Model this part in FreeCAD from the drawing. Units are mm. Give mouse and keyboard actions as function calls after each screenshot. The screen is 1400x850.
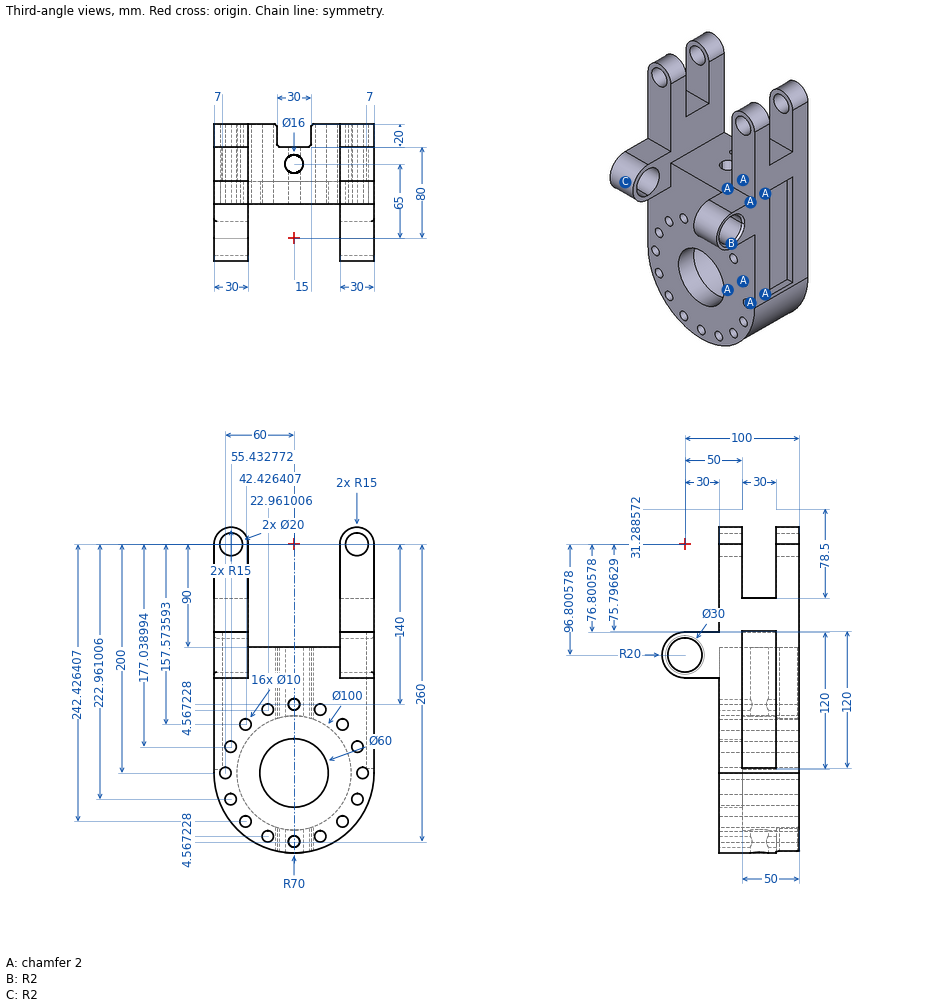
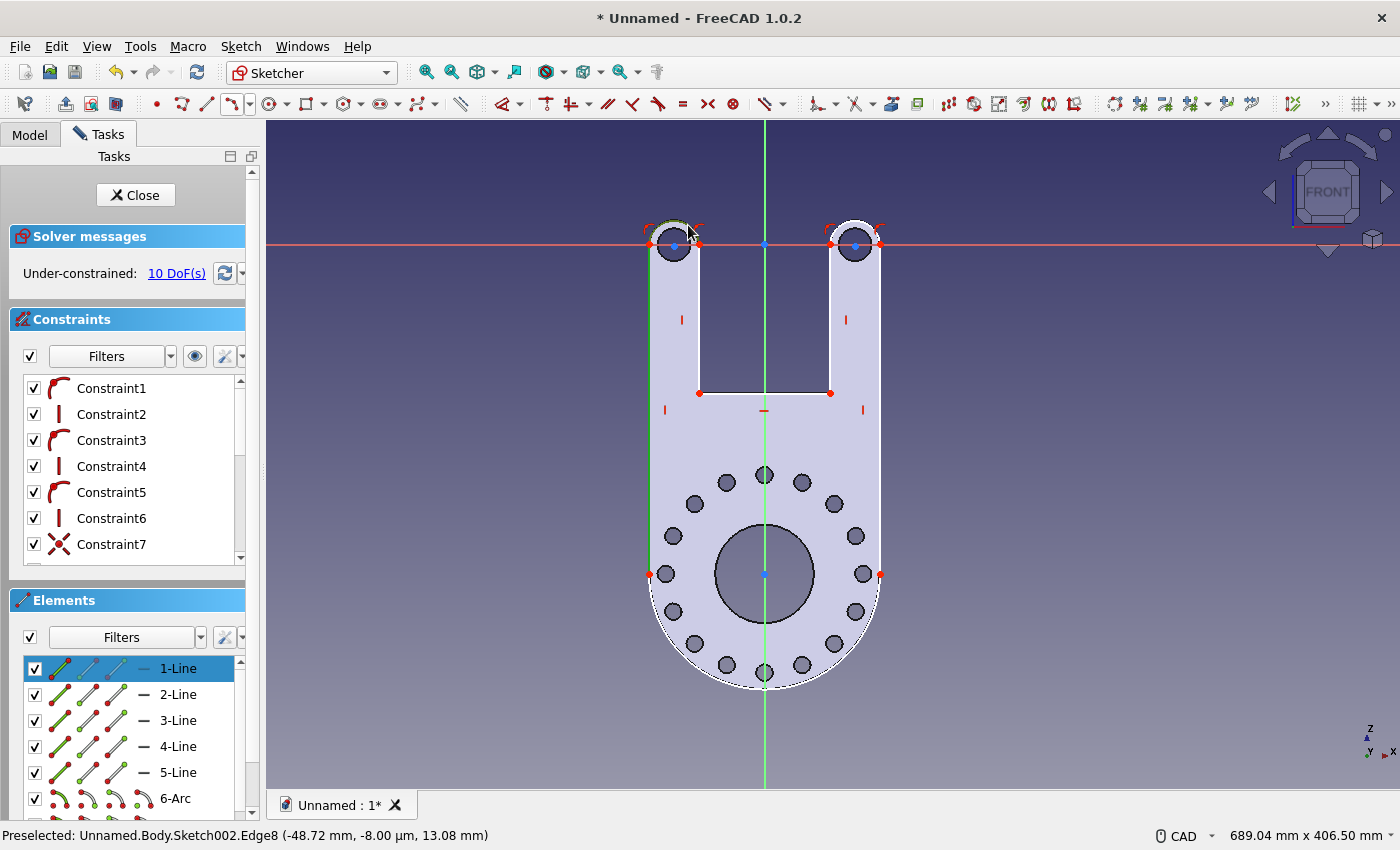
key(t)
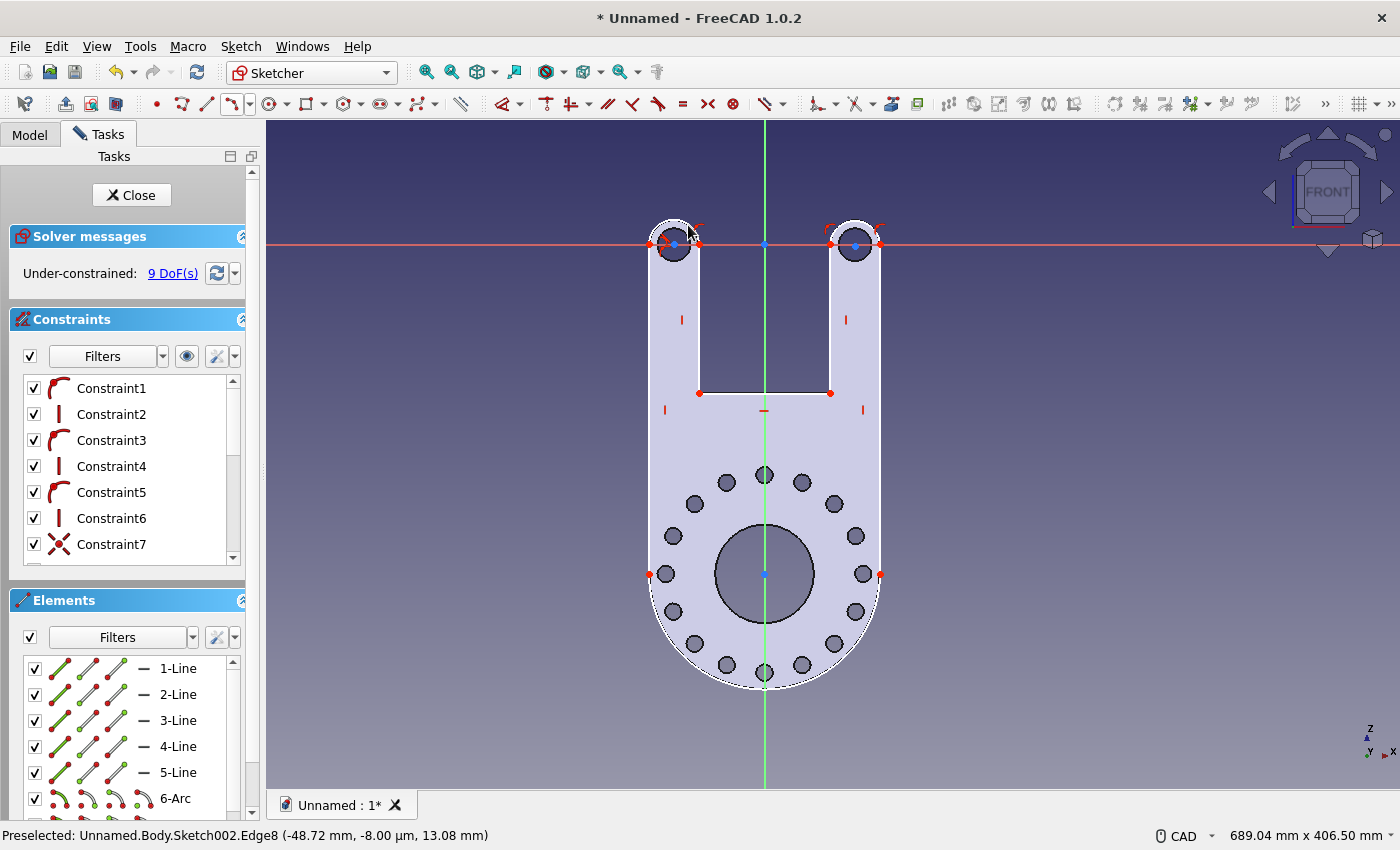
click(880, 476)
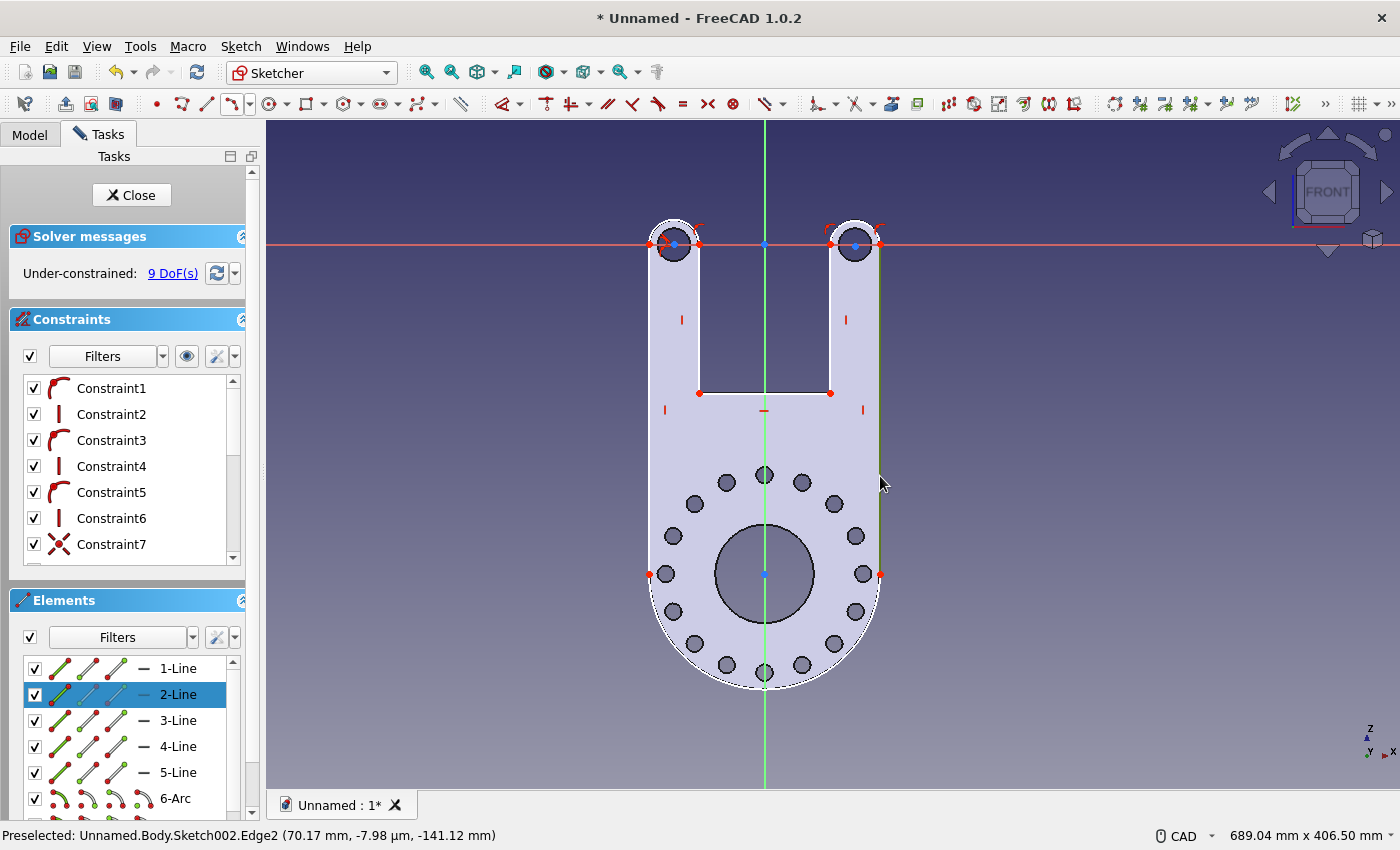
click(869, 225)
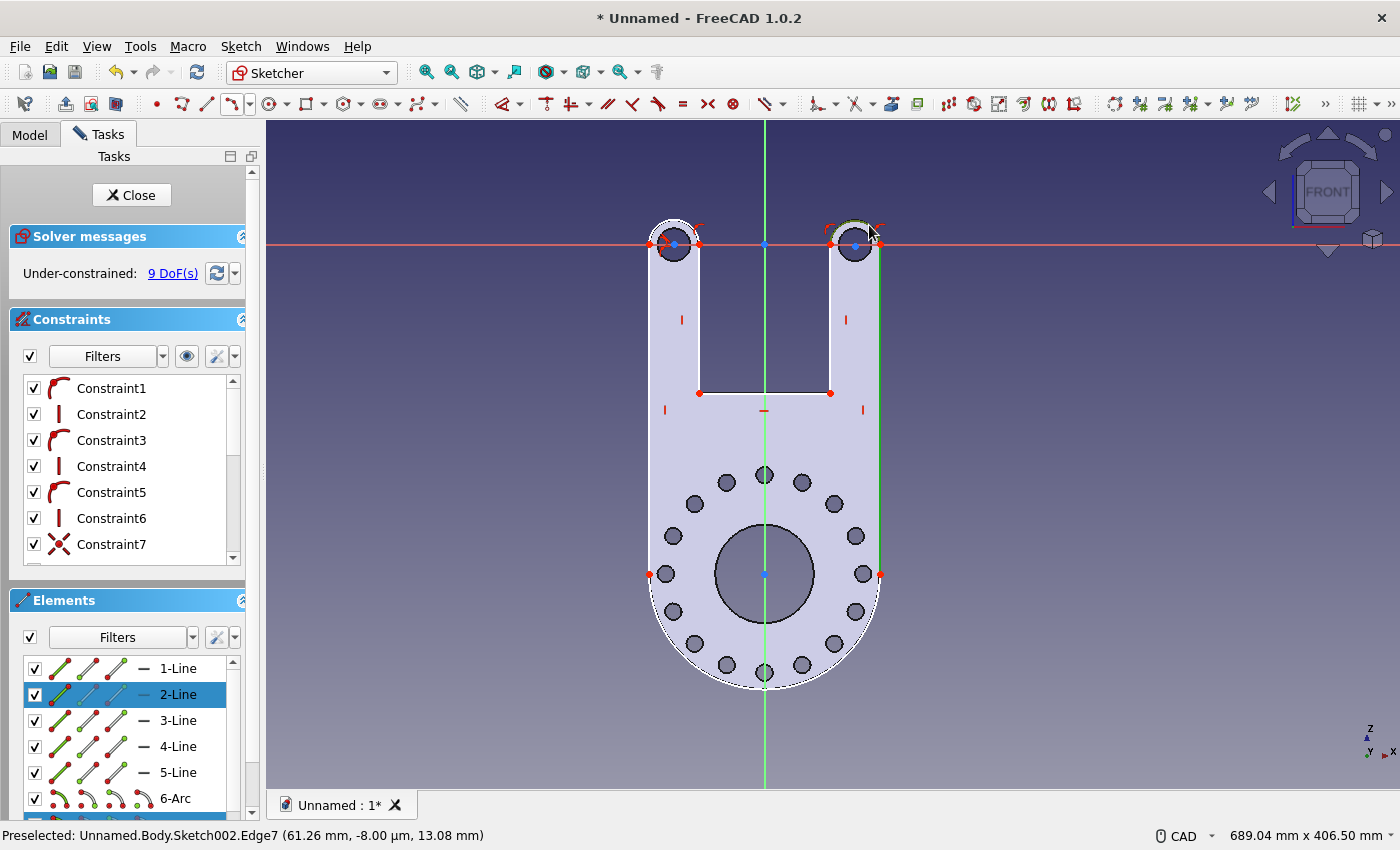
key(t)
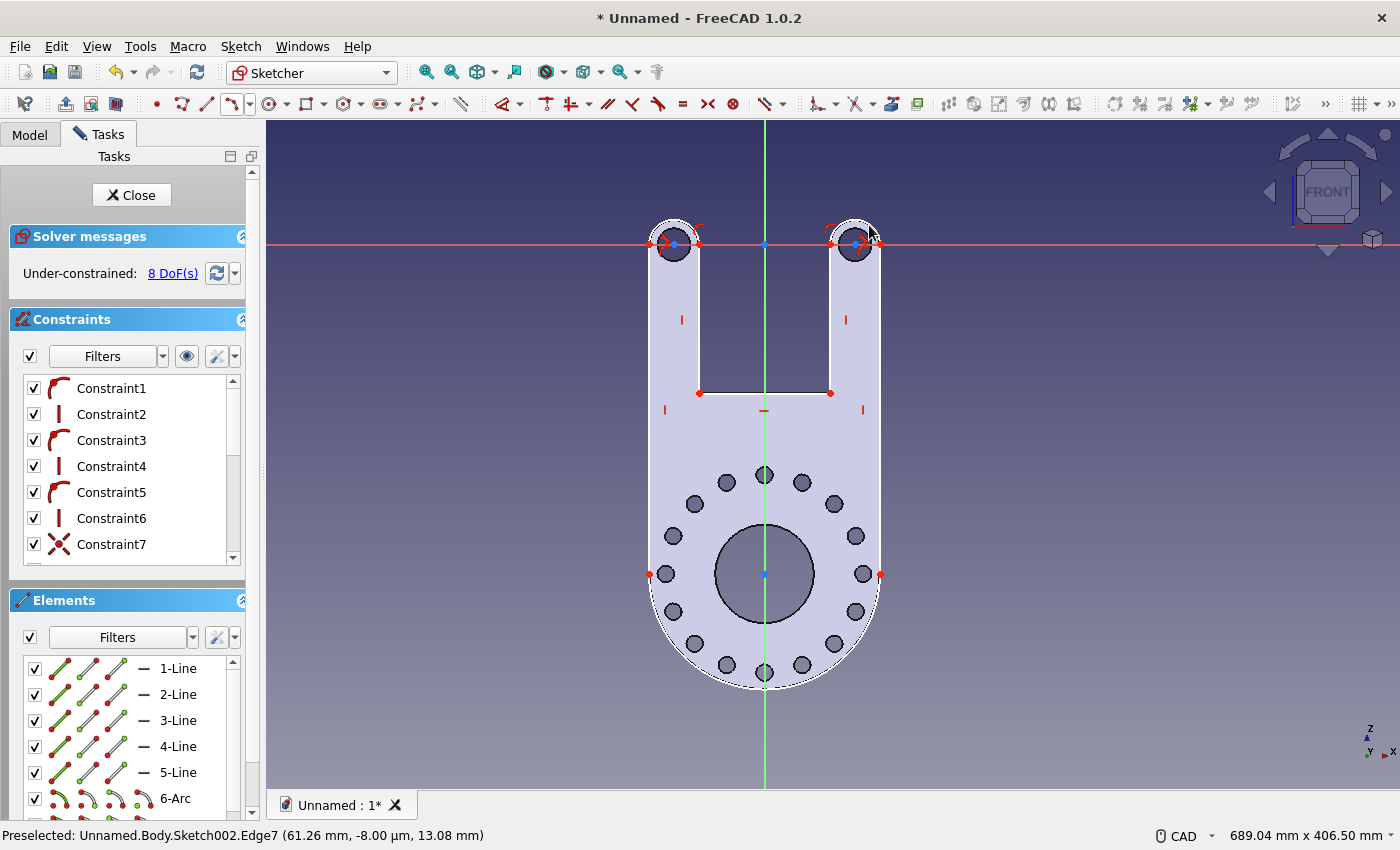
click(870, 225)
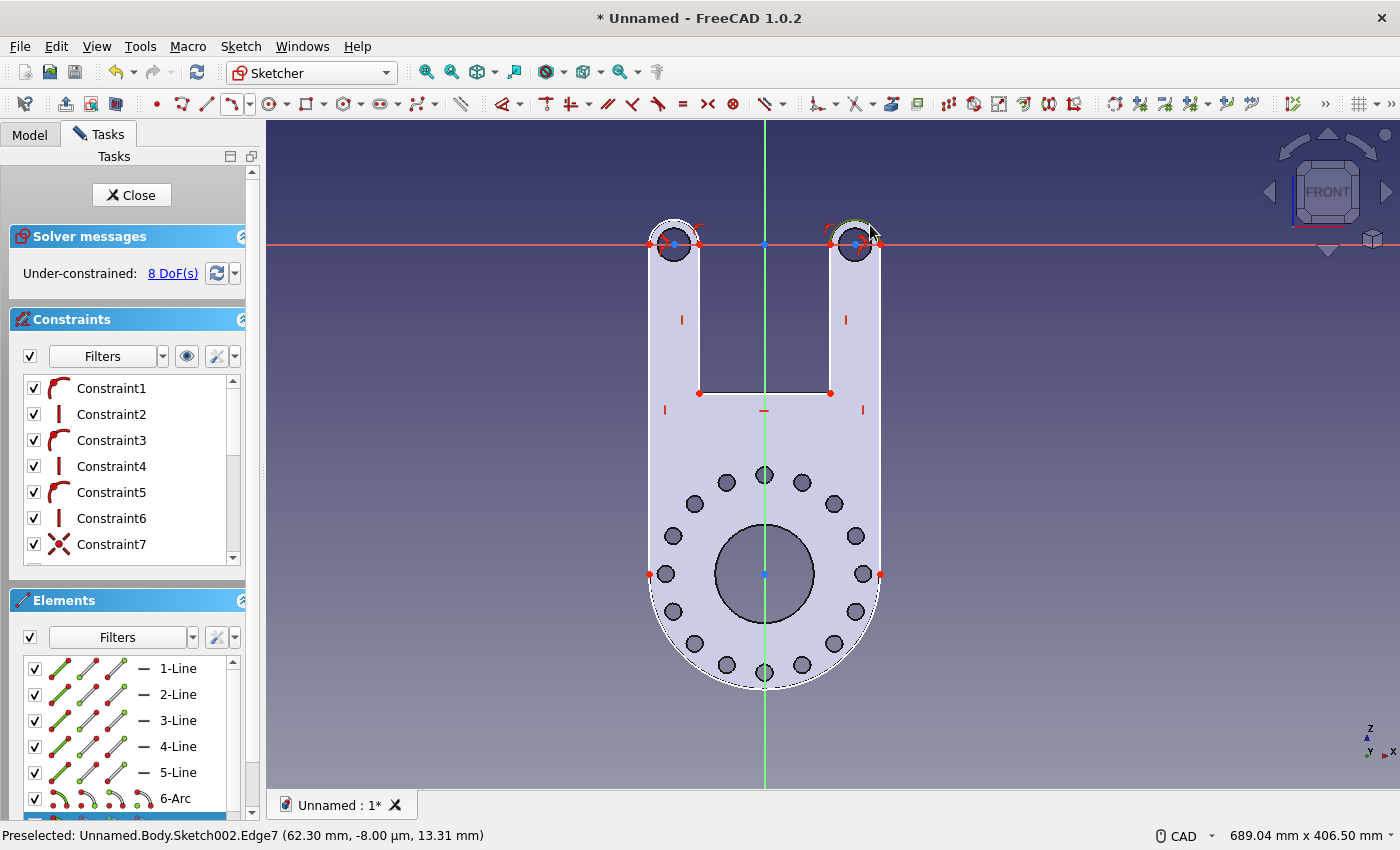
click(689, 225)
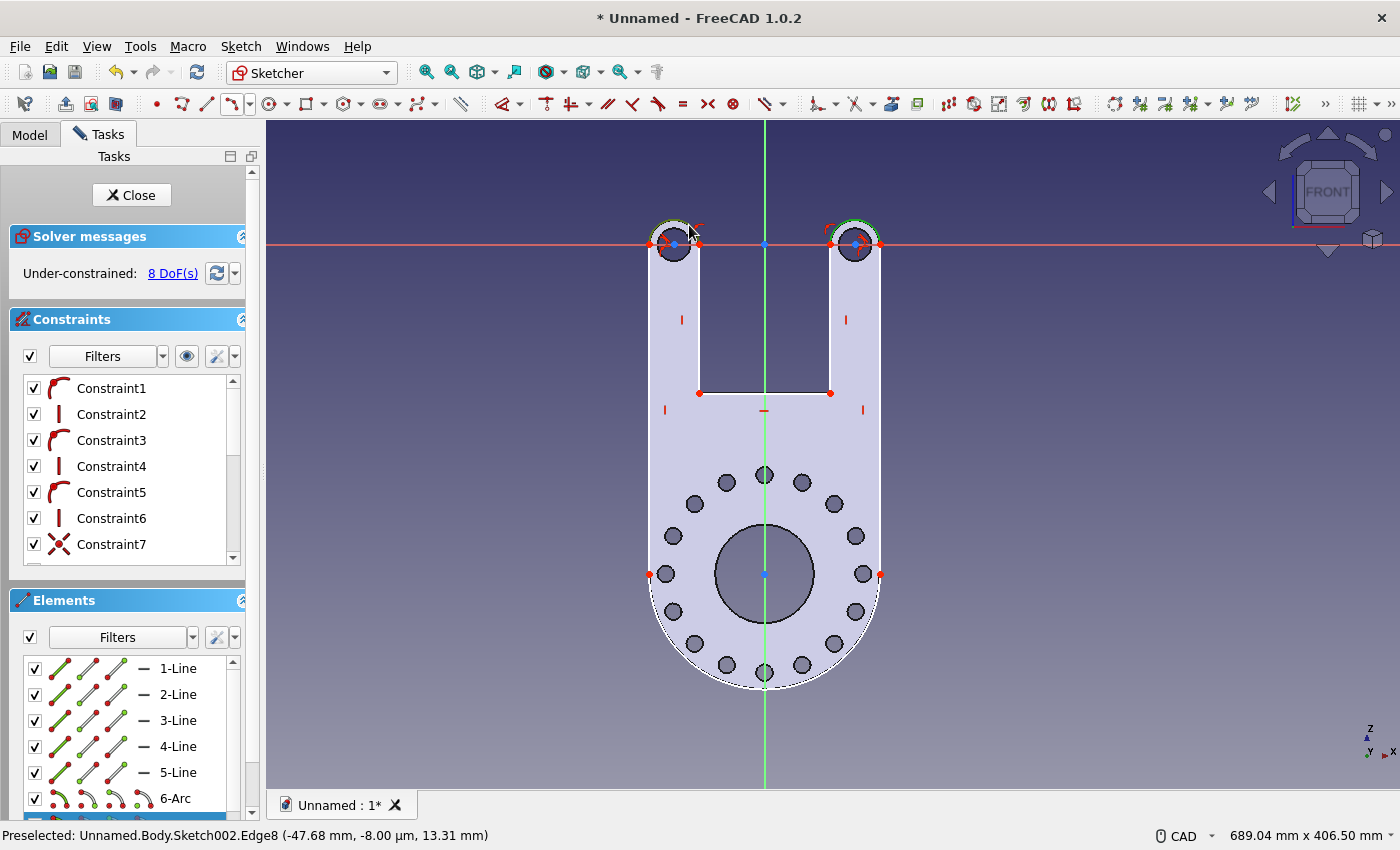
key(e)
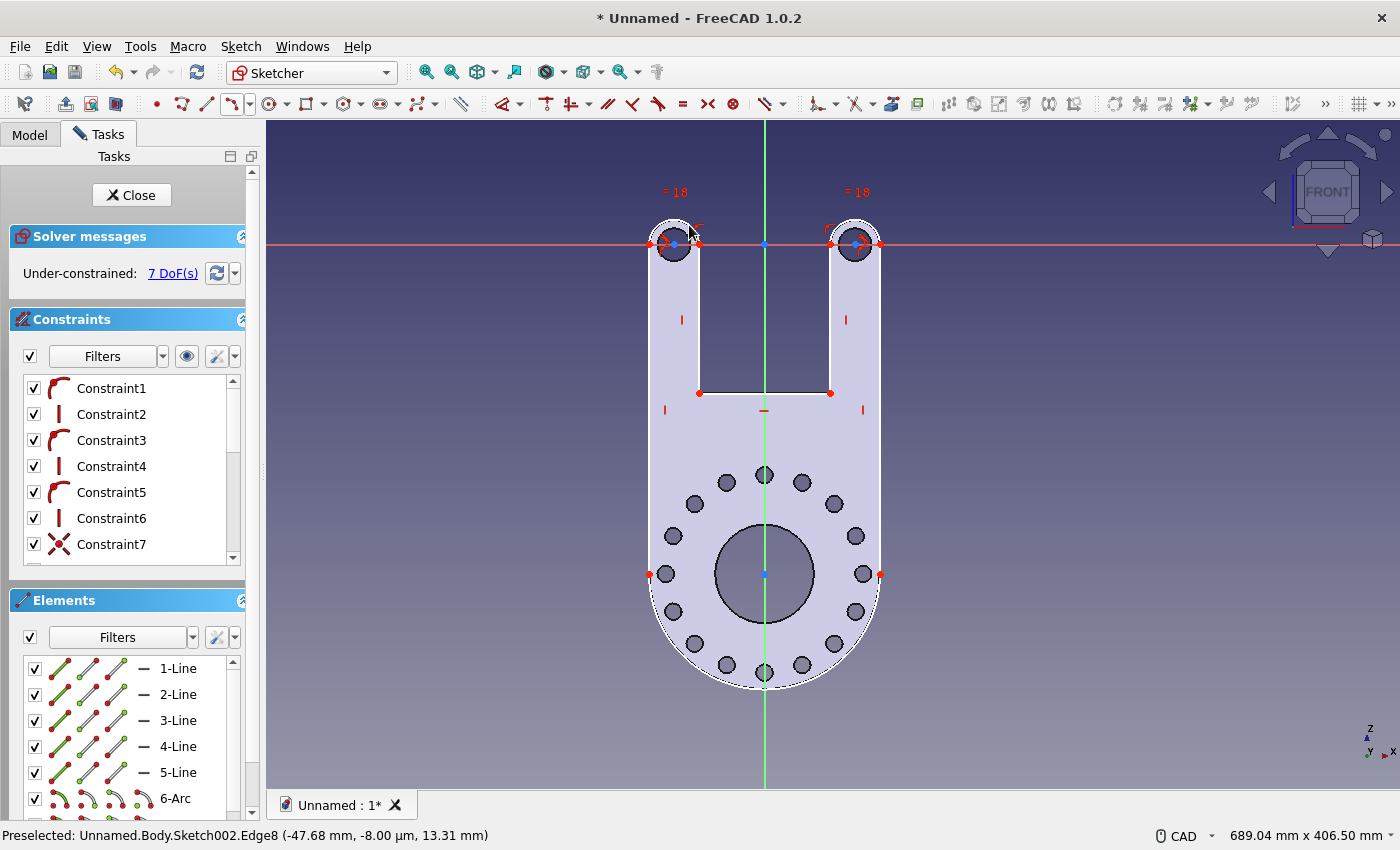
click(764, 574)